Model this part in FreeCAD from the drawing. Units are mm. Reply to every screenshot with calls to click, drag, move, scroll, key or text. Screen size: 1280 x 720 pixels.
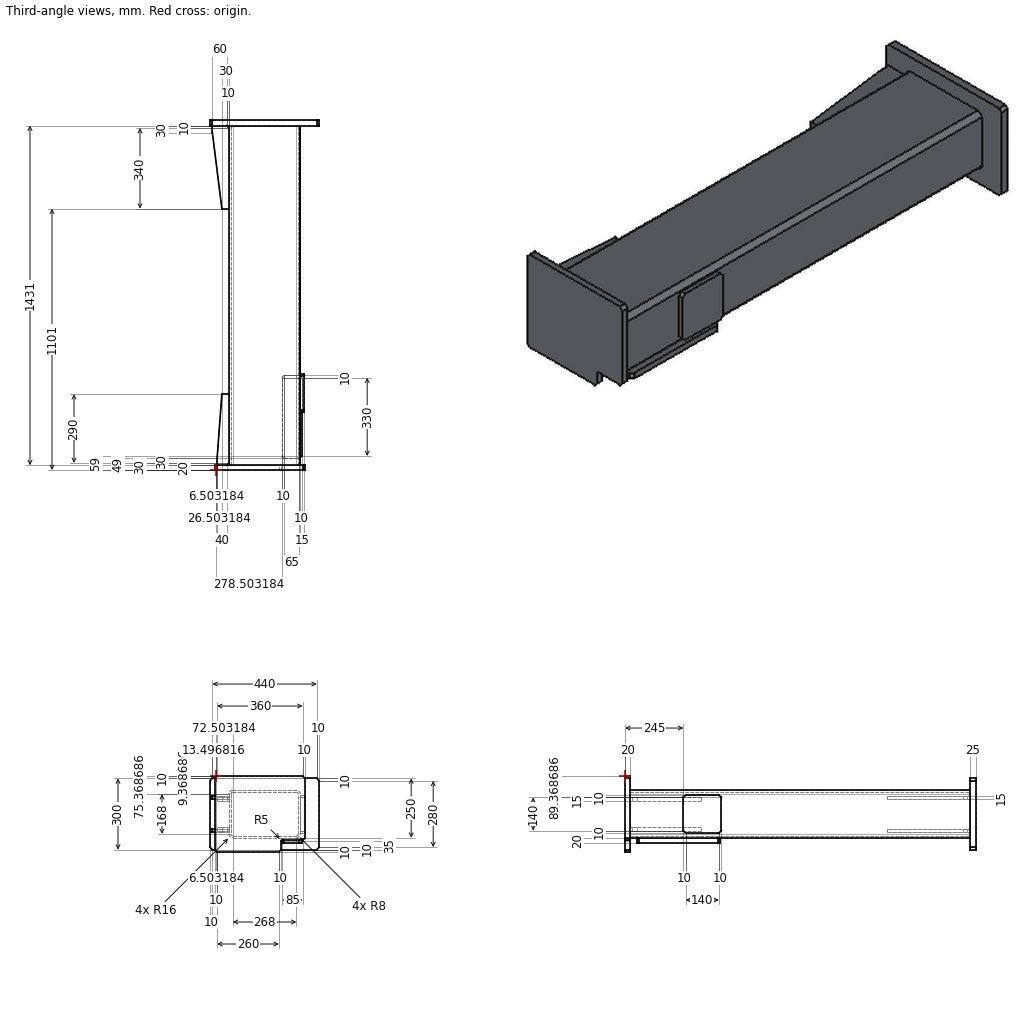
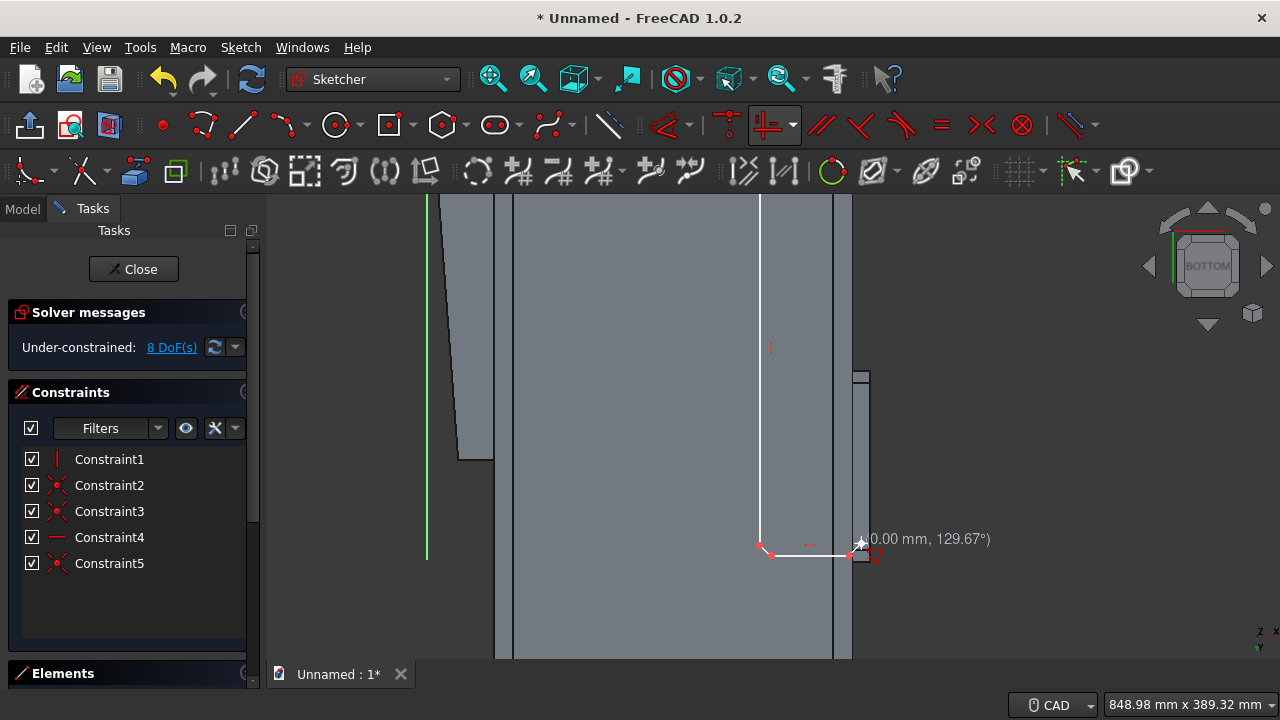
scroll(779, 561, down, 3)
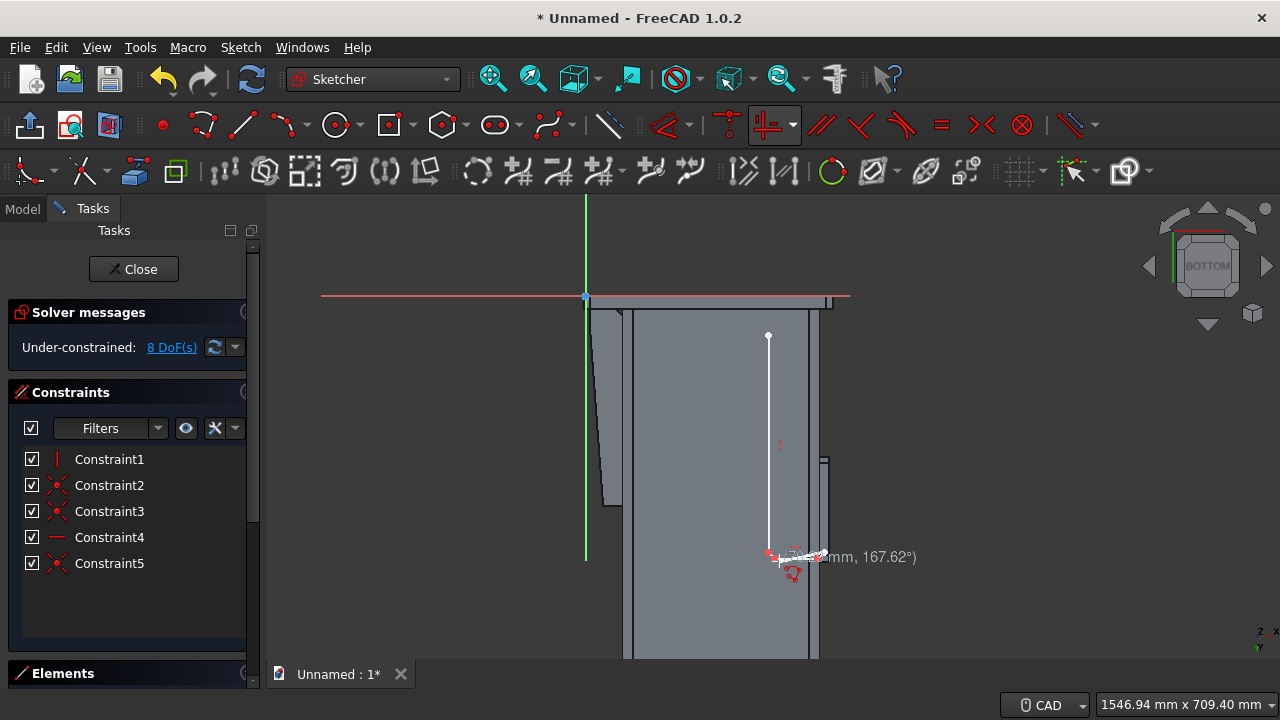
click(824, 335)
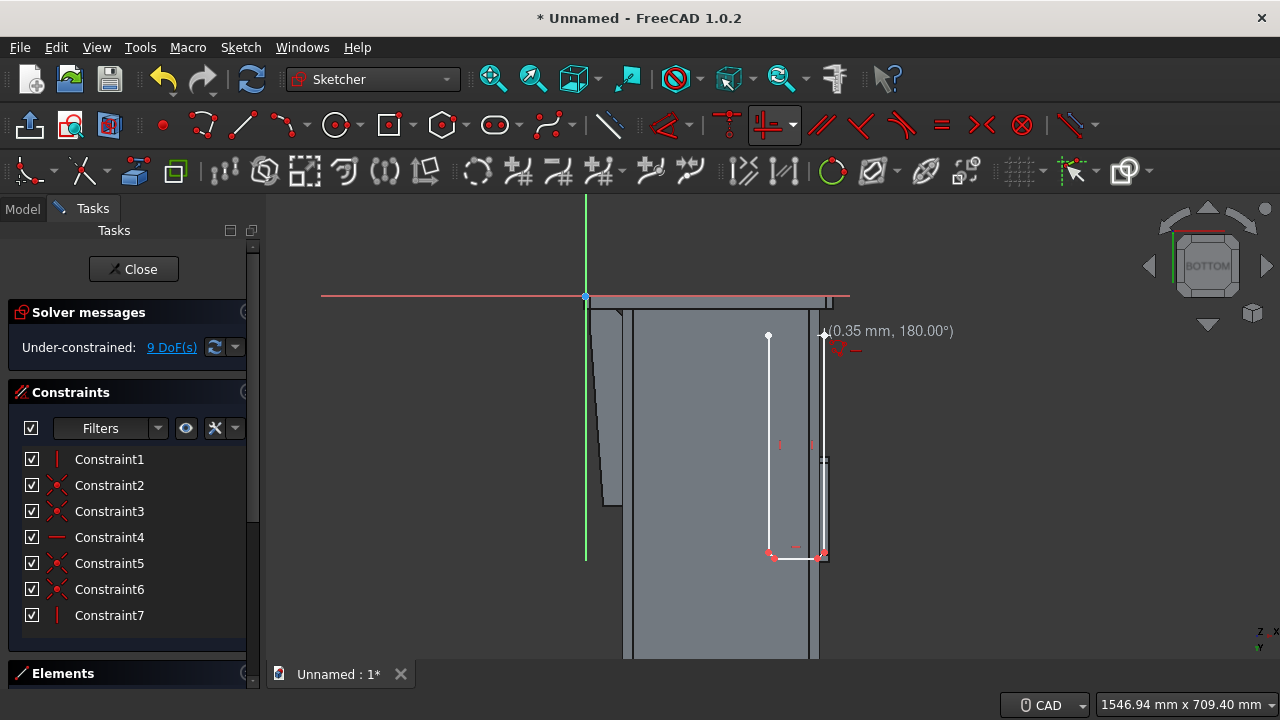
scroll(818, 328, up, 3)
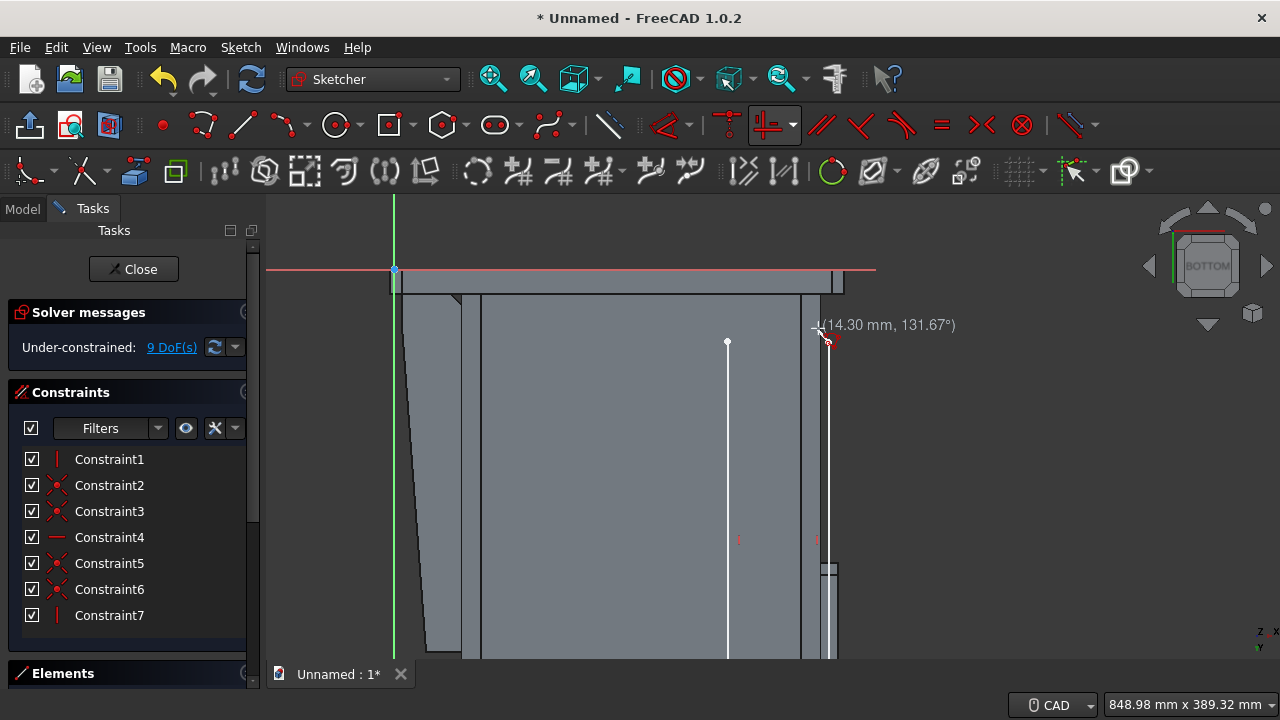
click(817, 329)
click(739, 329)
click(728, 342)
key(Escape)
key(Escape)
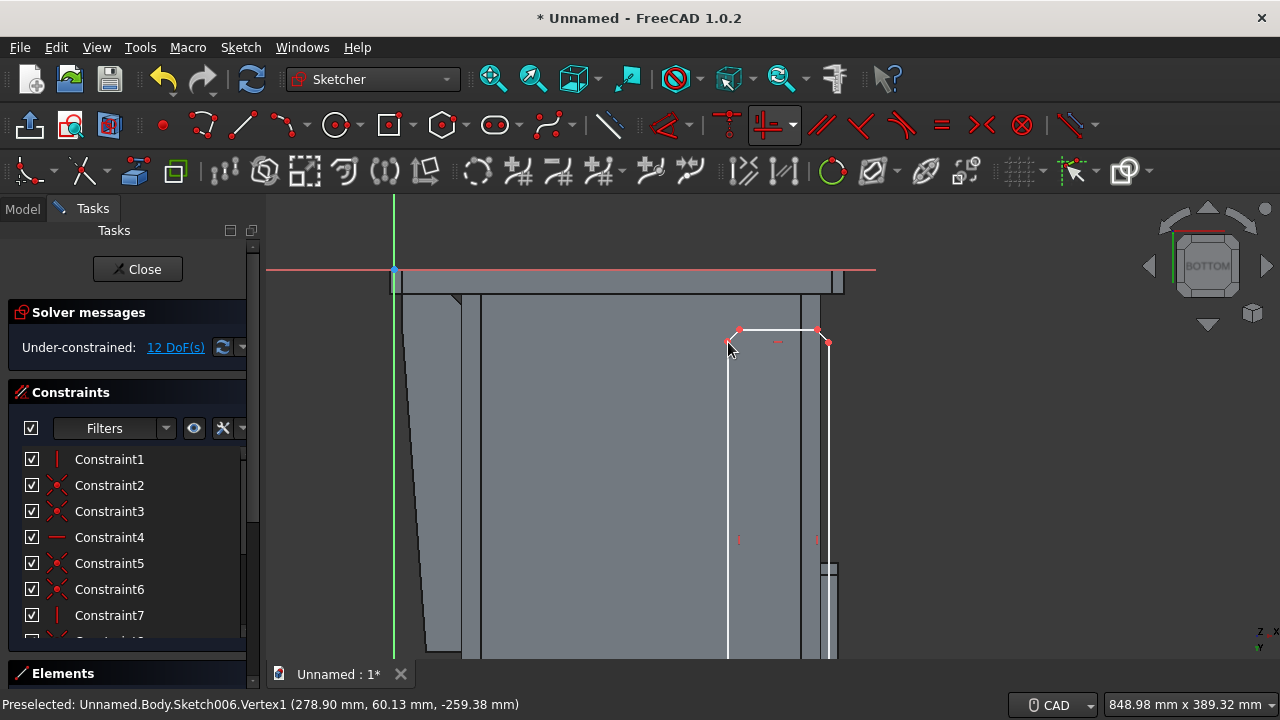
click(664, 126)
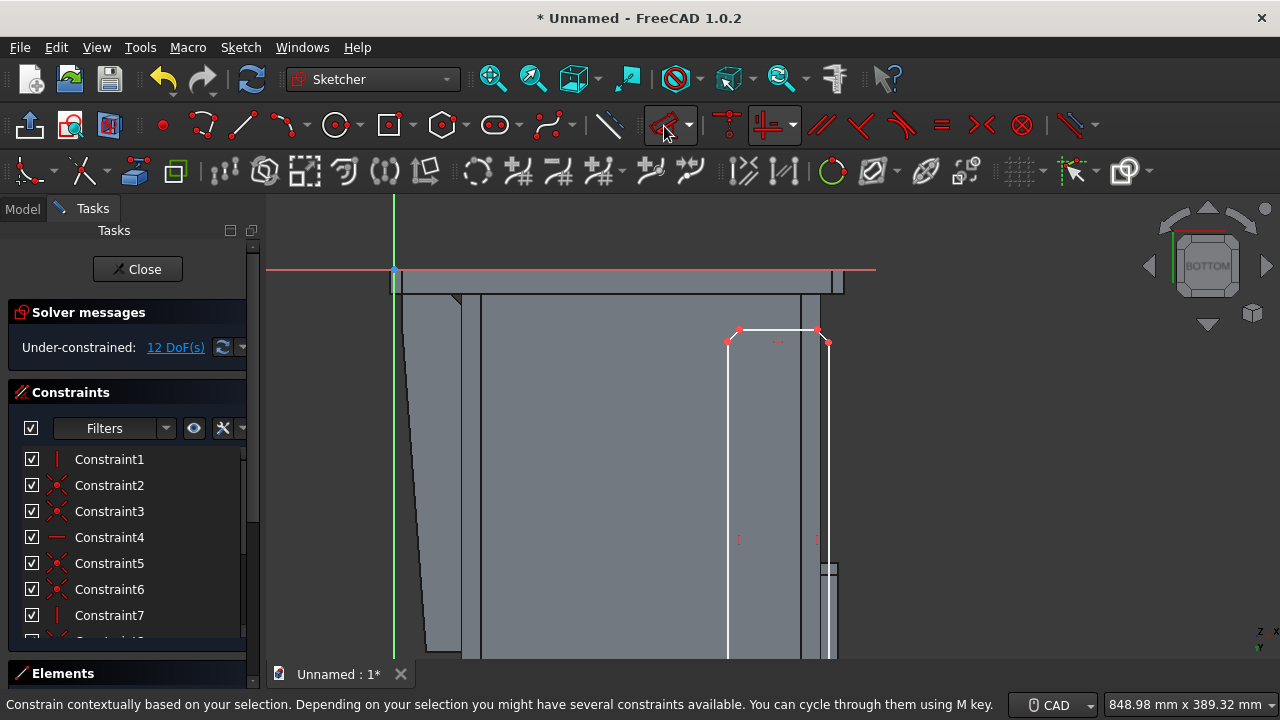
scroll(818, 327, down, 3)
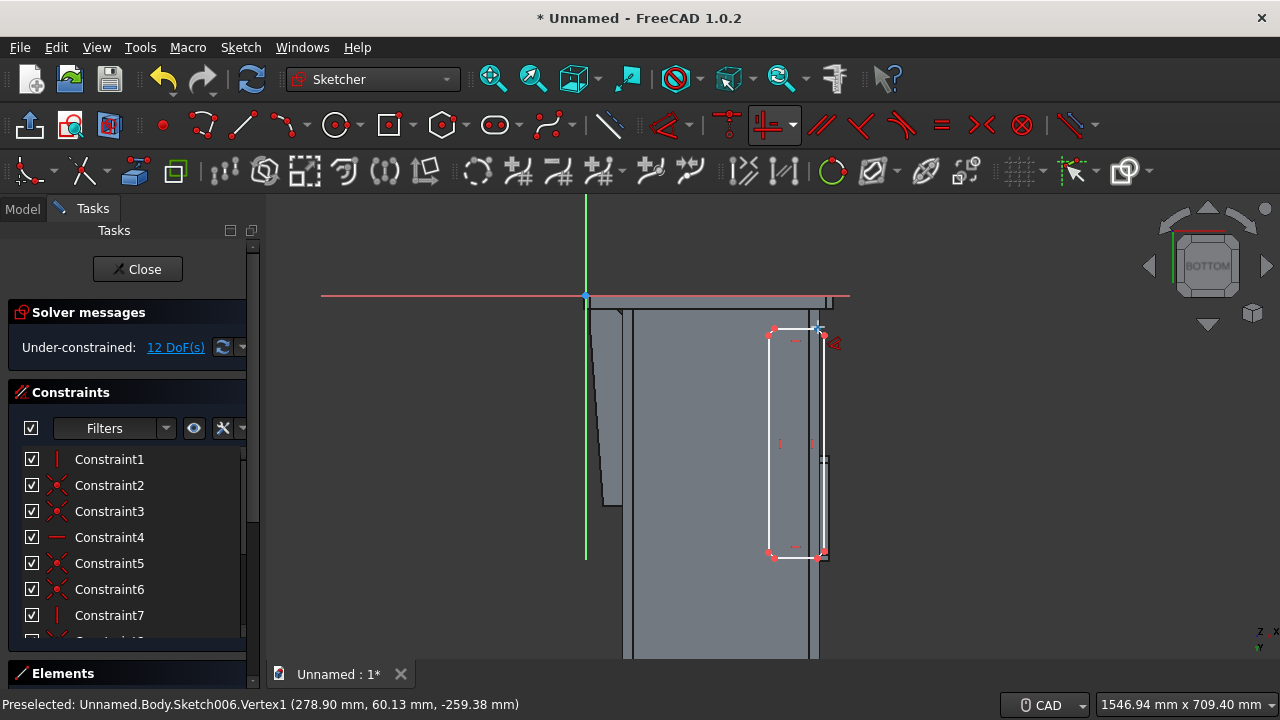
click(788, 558)
click(796, 592)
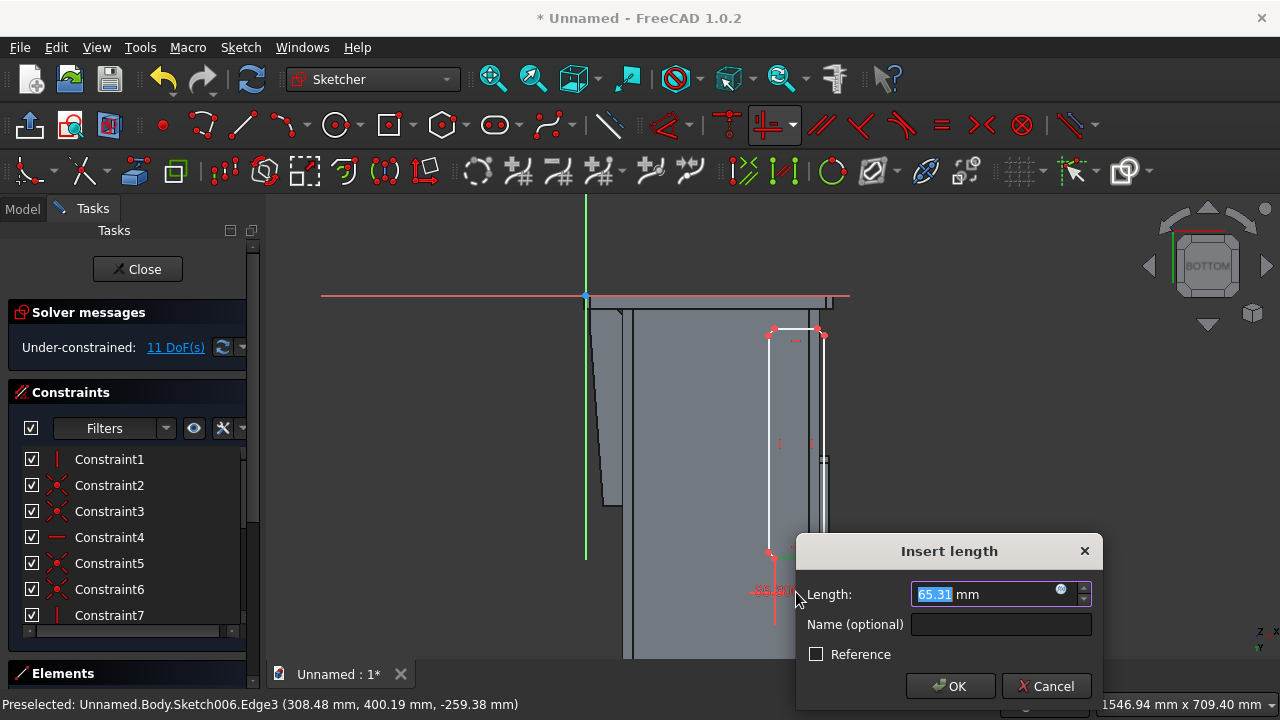
text(65)
key(Return)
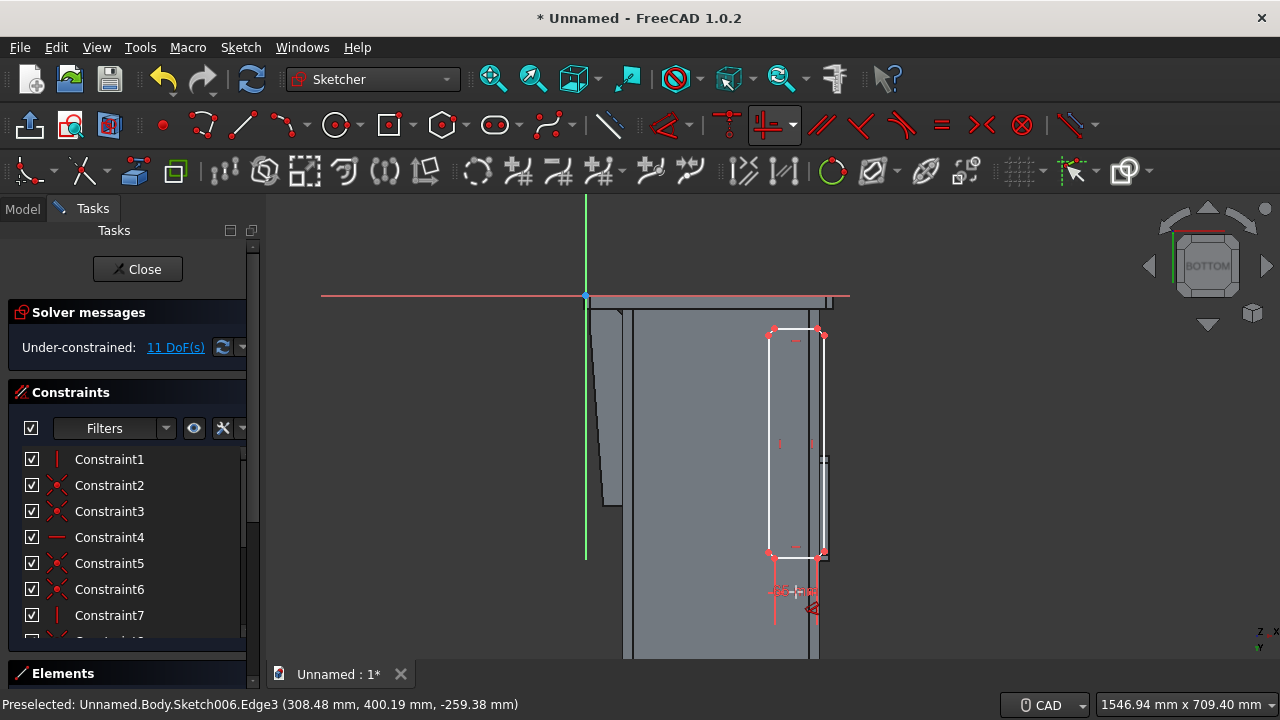
click(805, 329)
click(796, 363)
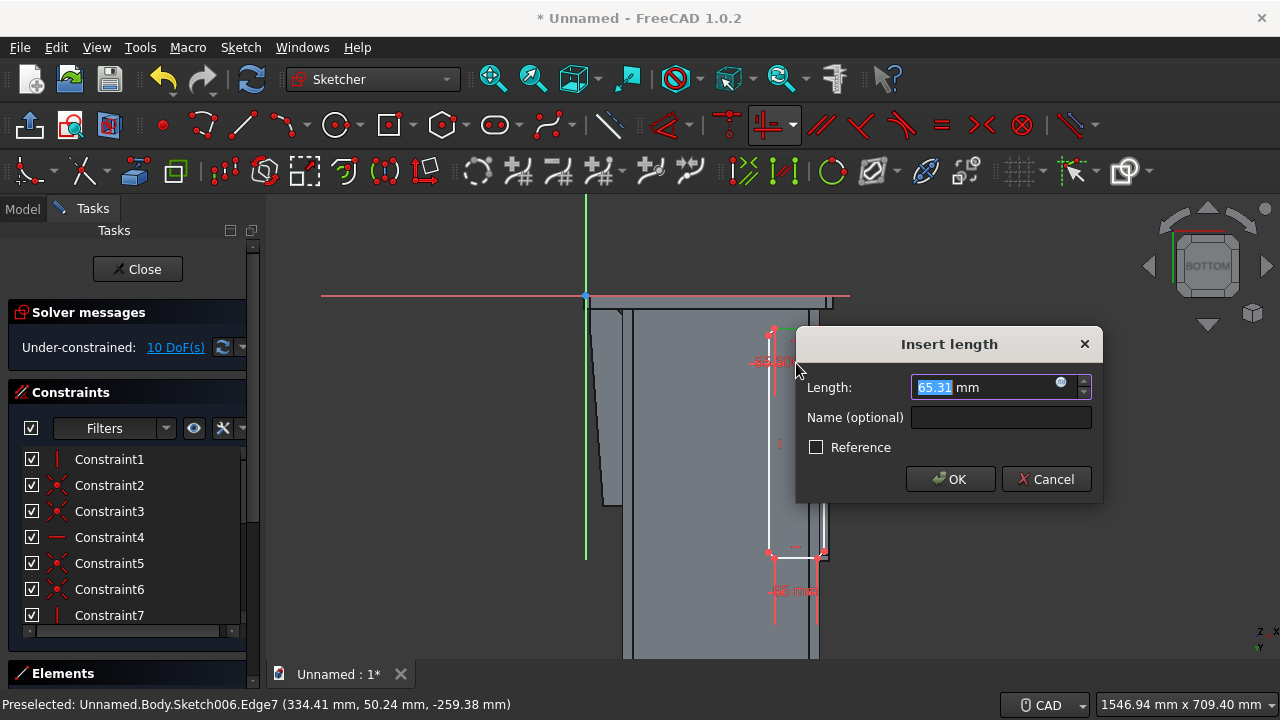
text(65)
key(Return)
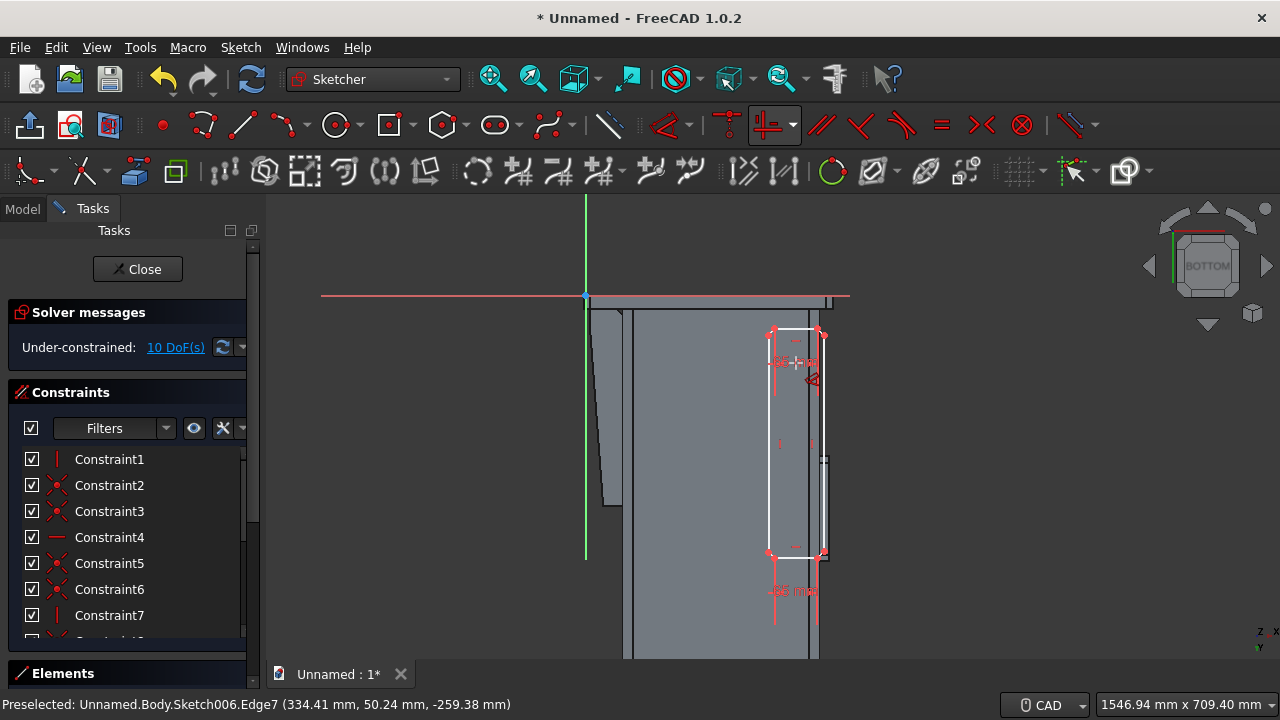
click(769, 400)
click(803, 444)